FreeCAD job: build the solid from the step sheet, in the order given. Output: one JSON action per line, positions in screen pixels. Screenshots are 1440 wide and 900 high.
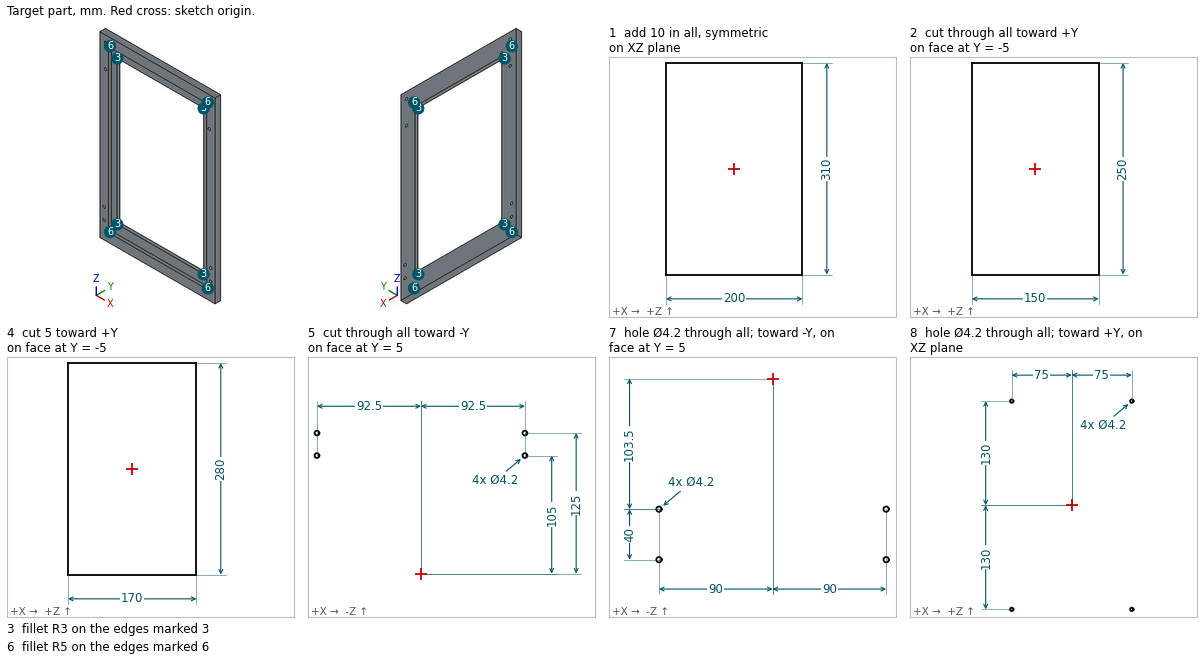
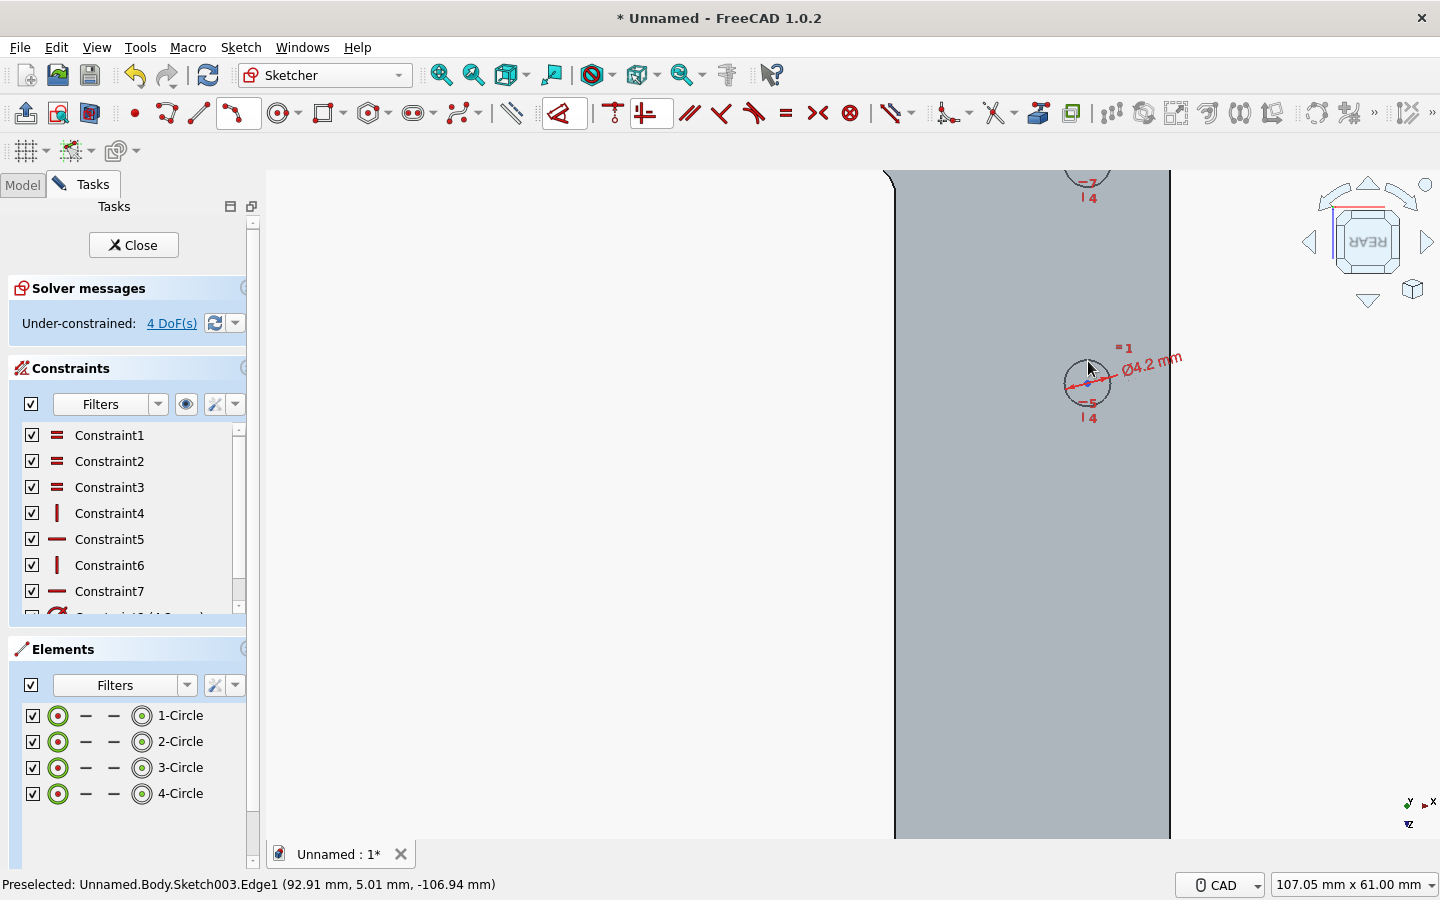
{"action": "left_click", "coordinate": [1088, 383]}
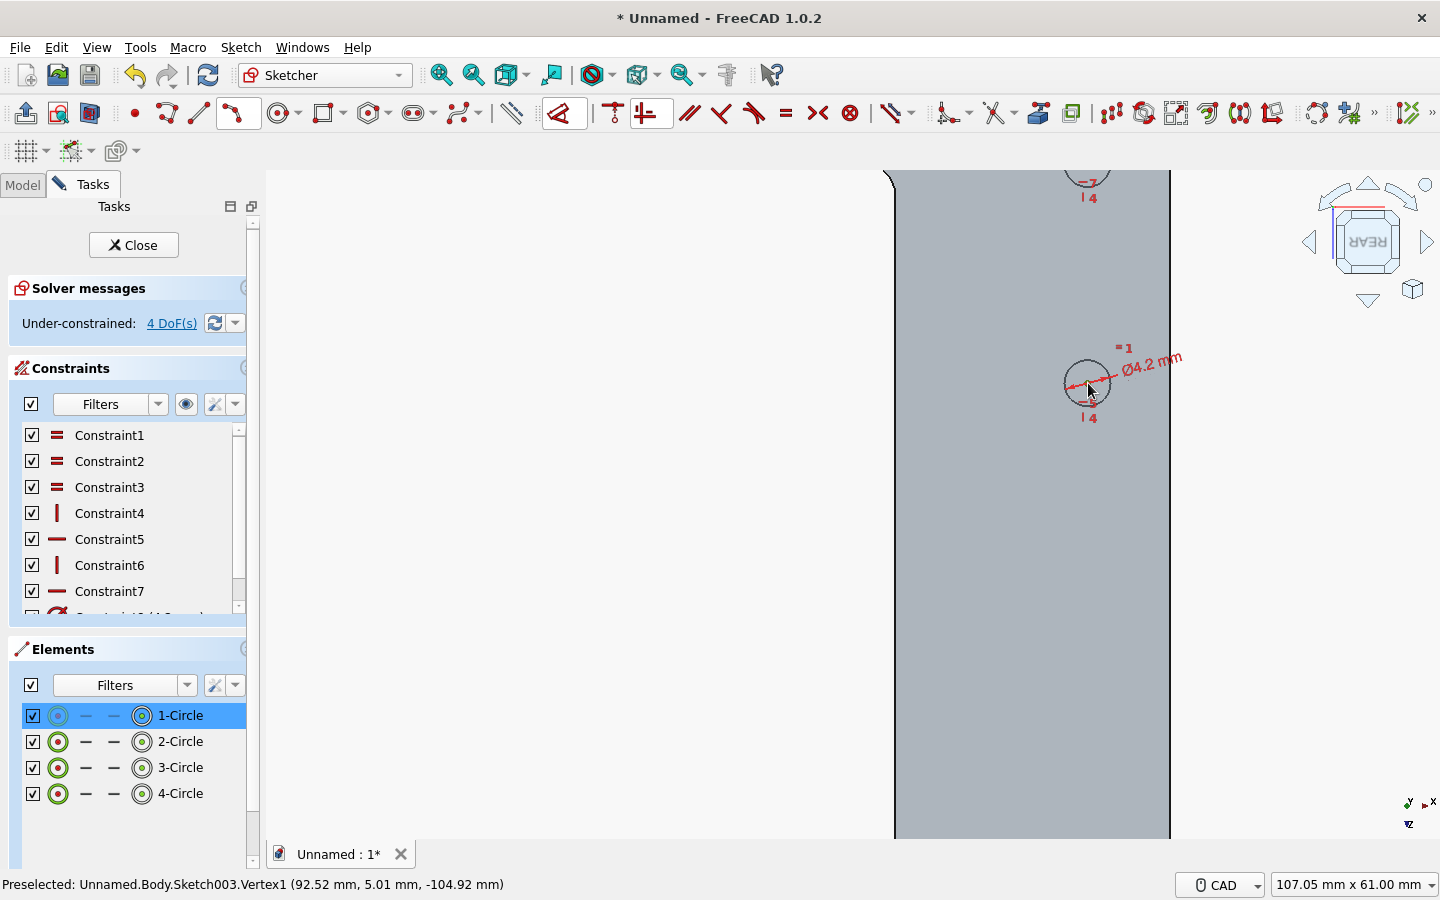
{"action": "key", "text": "i"}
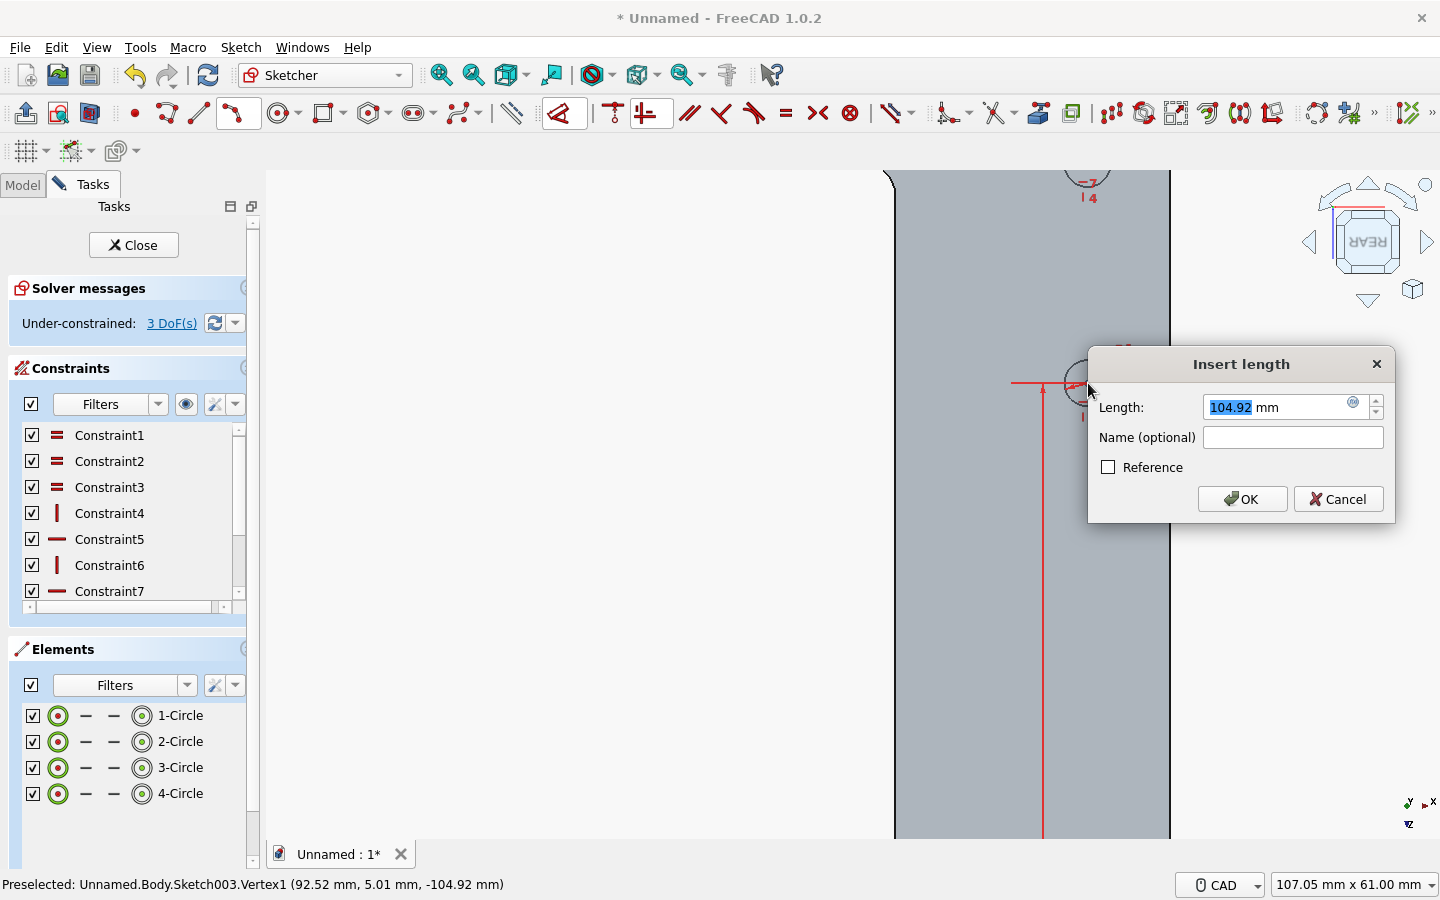
{"action": "type", "text": "105"}
{"action": "key", "text": "Return"}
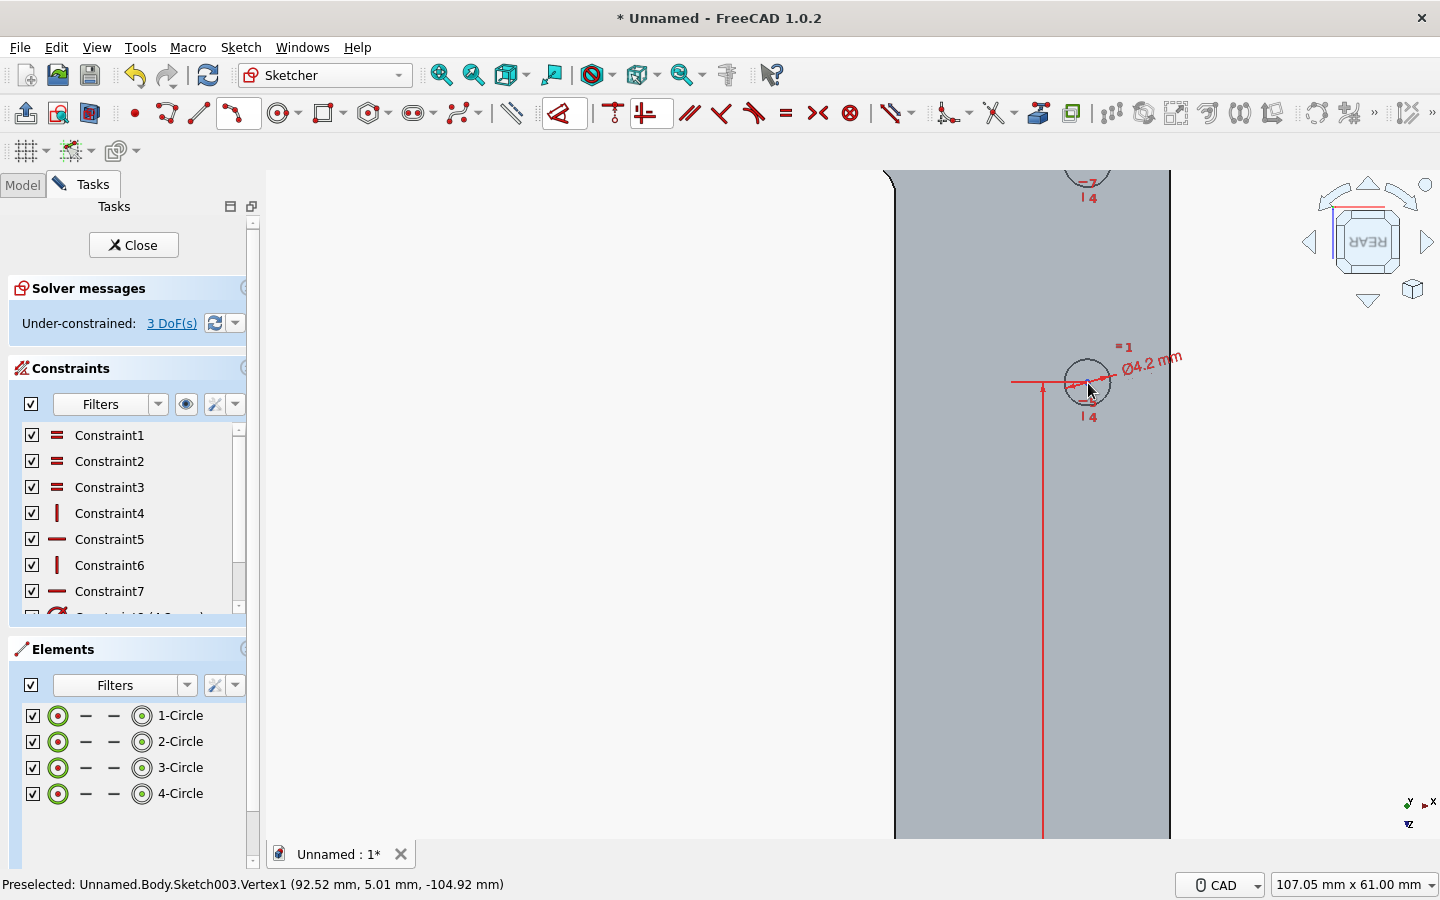
{"action": "scroll", "coordinate": [1091, 361], "scroll_direction": "down", "scroll_amount": 6}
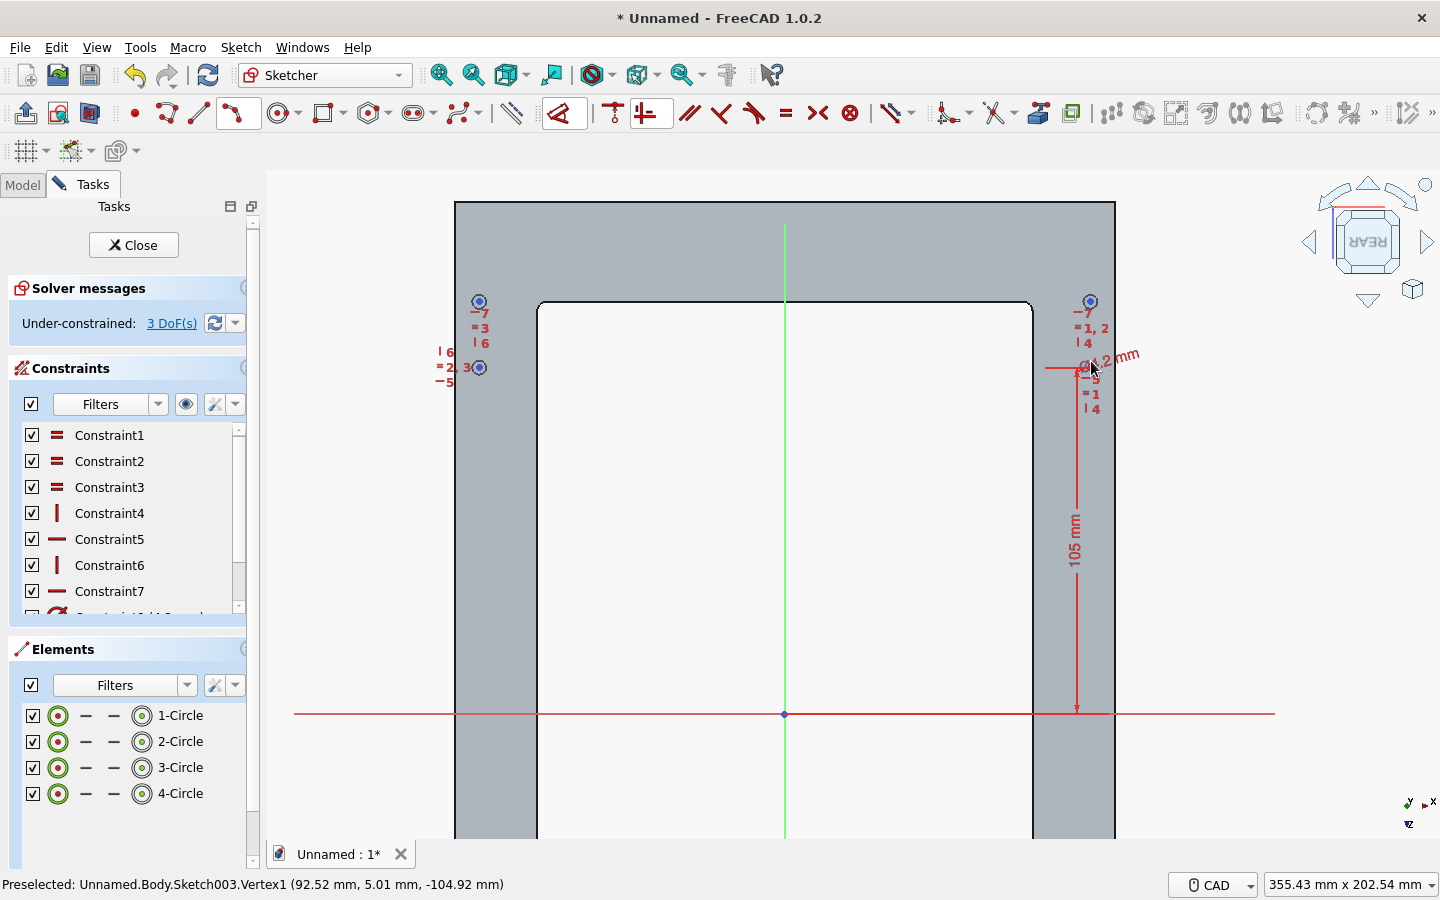
{"action": "left_click", "coordinate": [1090, 302]}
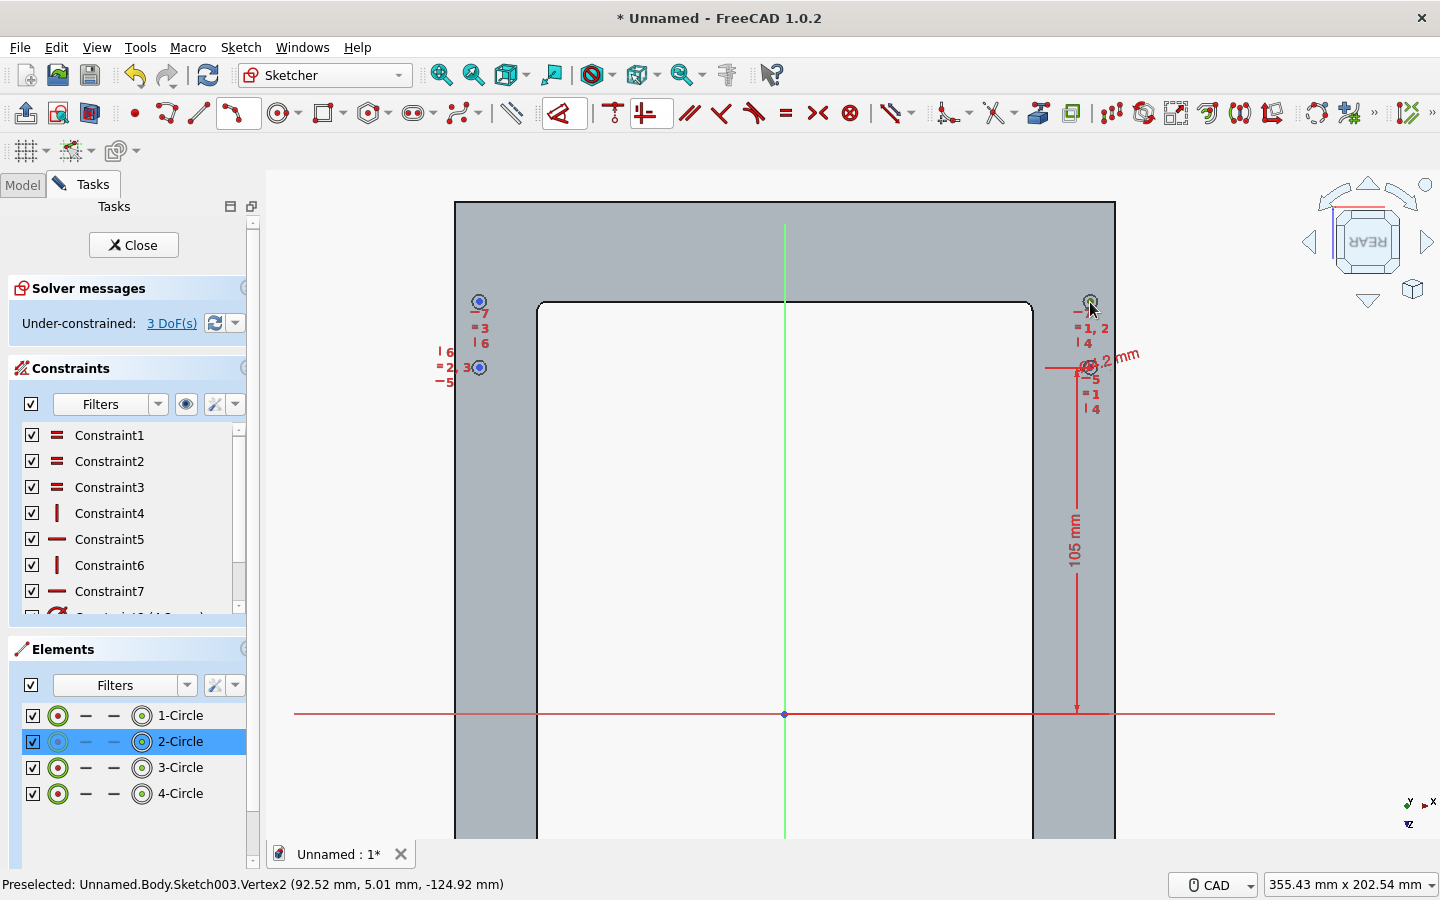
{"action": "key", "text": "i"}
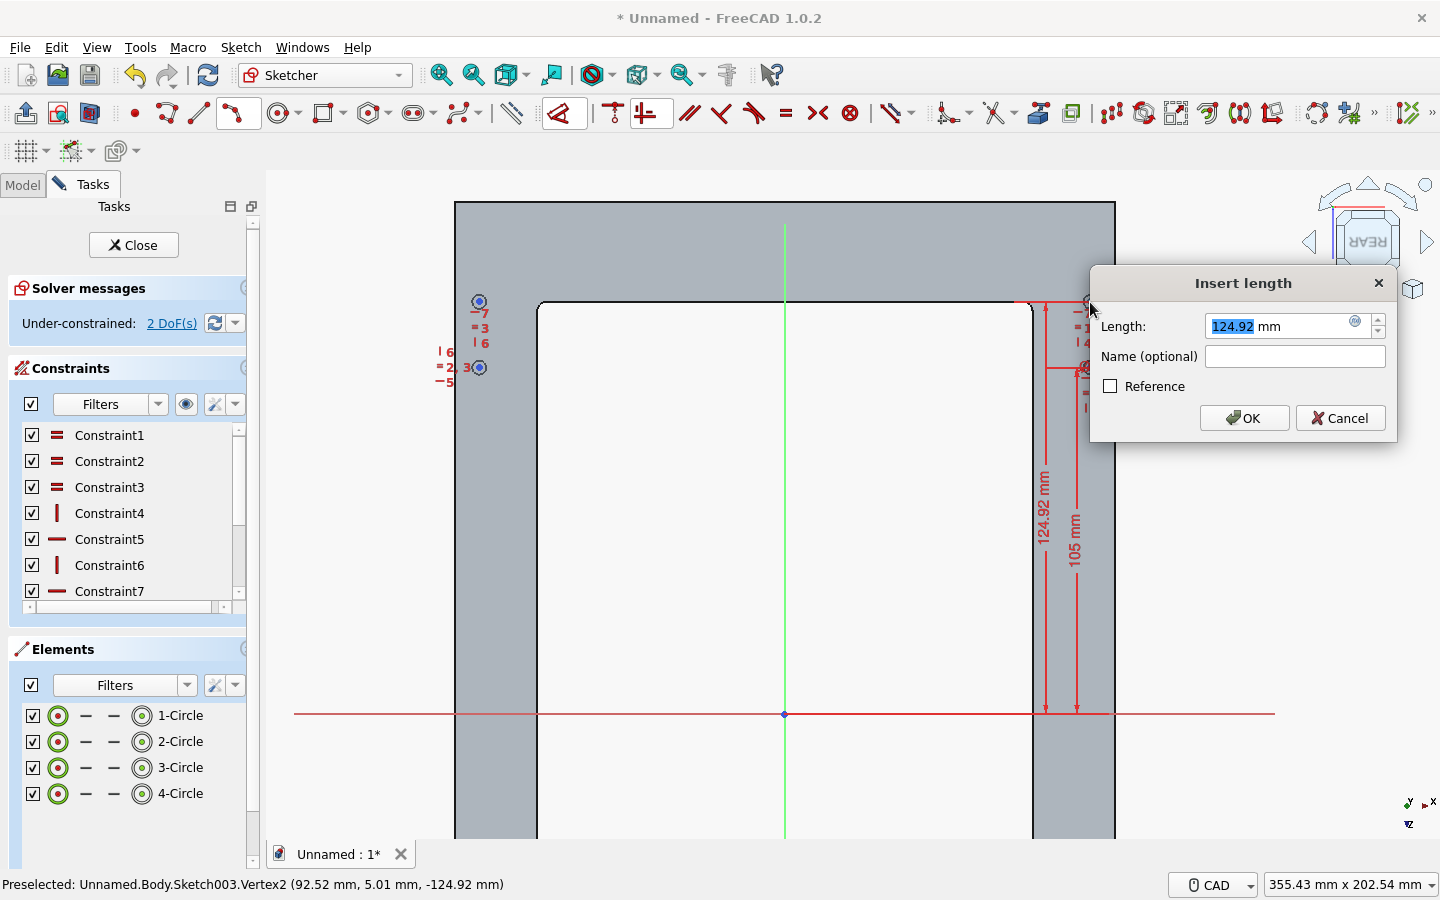
{"action": "type", "text": "125"}
{"action": "key", "text": "Return"}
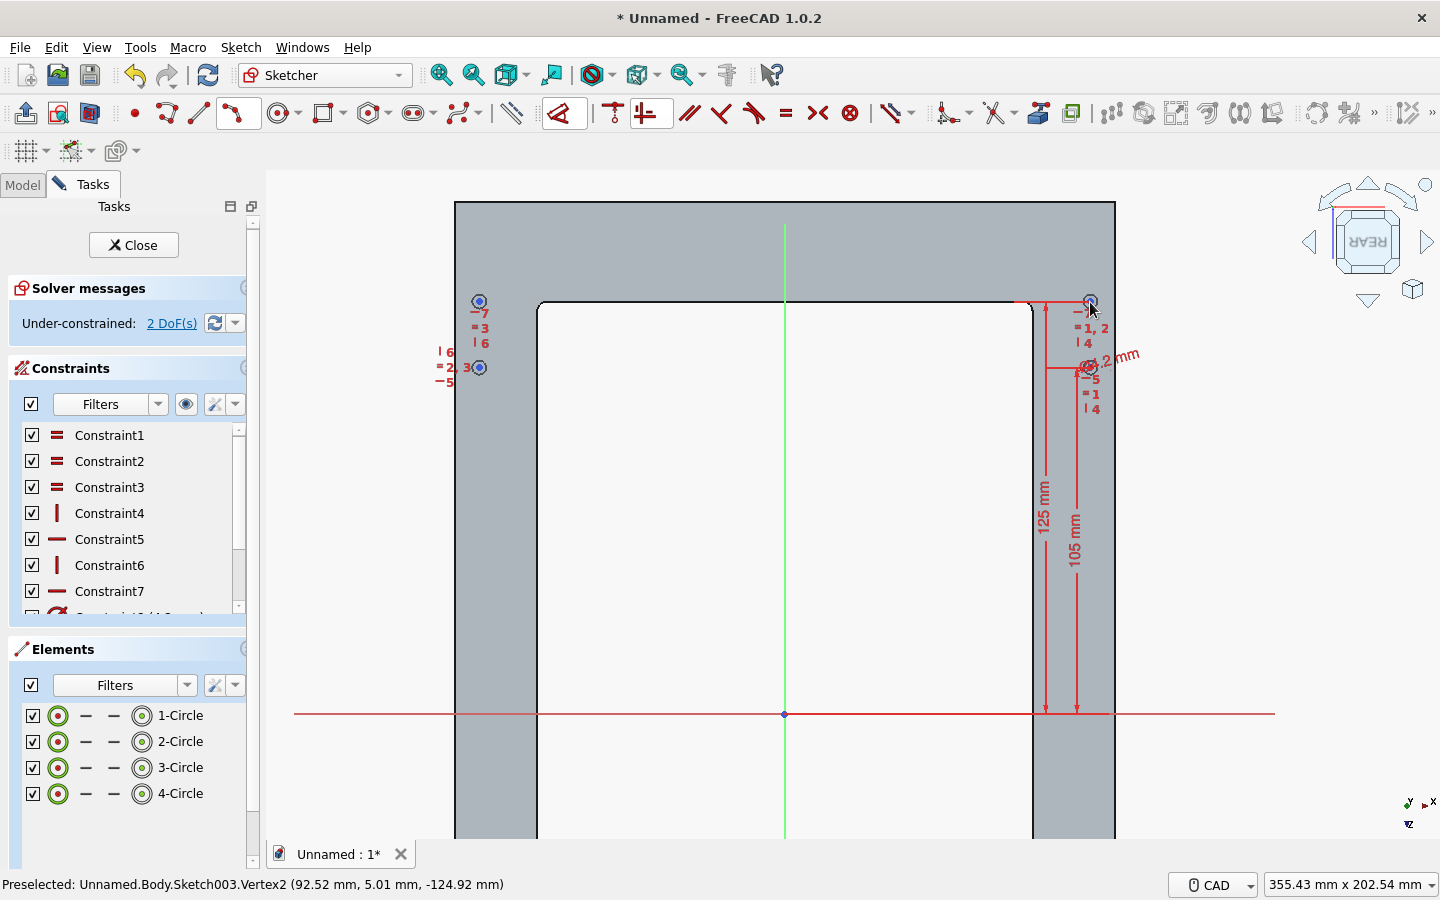
{"action": "left_click", "coordinate": [1090, 368]}